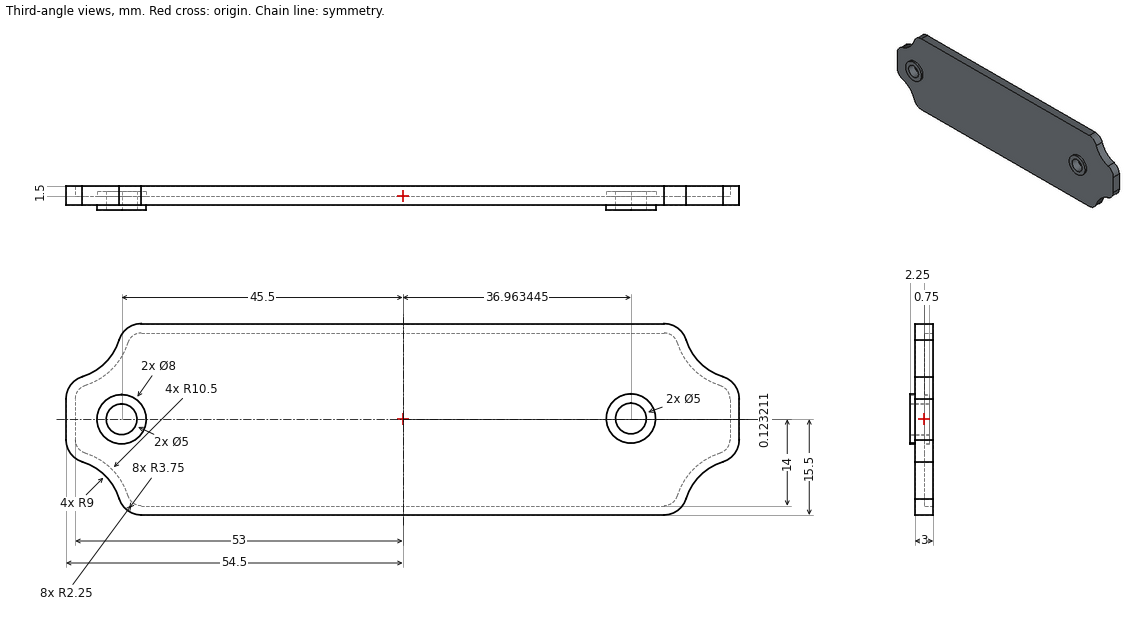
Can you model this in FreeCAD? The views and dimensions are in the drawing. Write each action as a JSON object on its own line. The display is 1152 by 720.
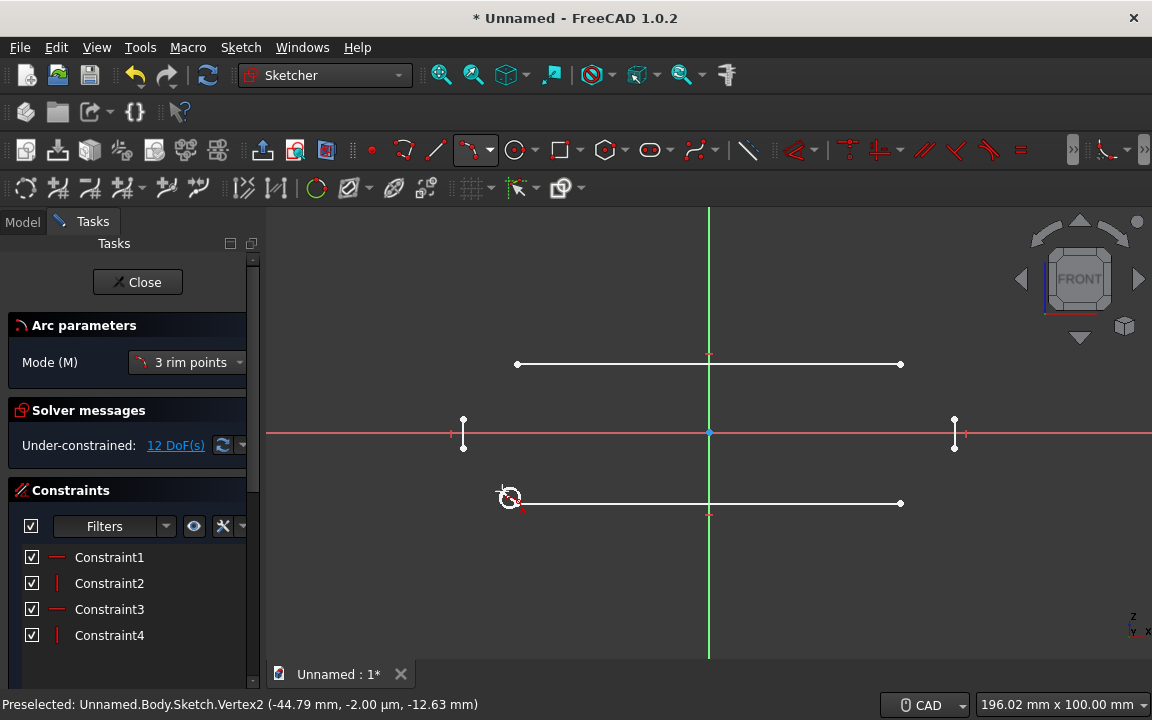
{"action": "scroll", "coordinate": [508, 500], "scroll_direction": "up", "scroll_amount": 8}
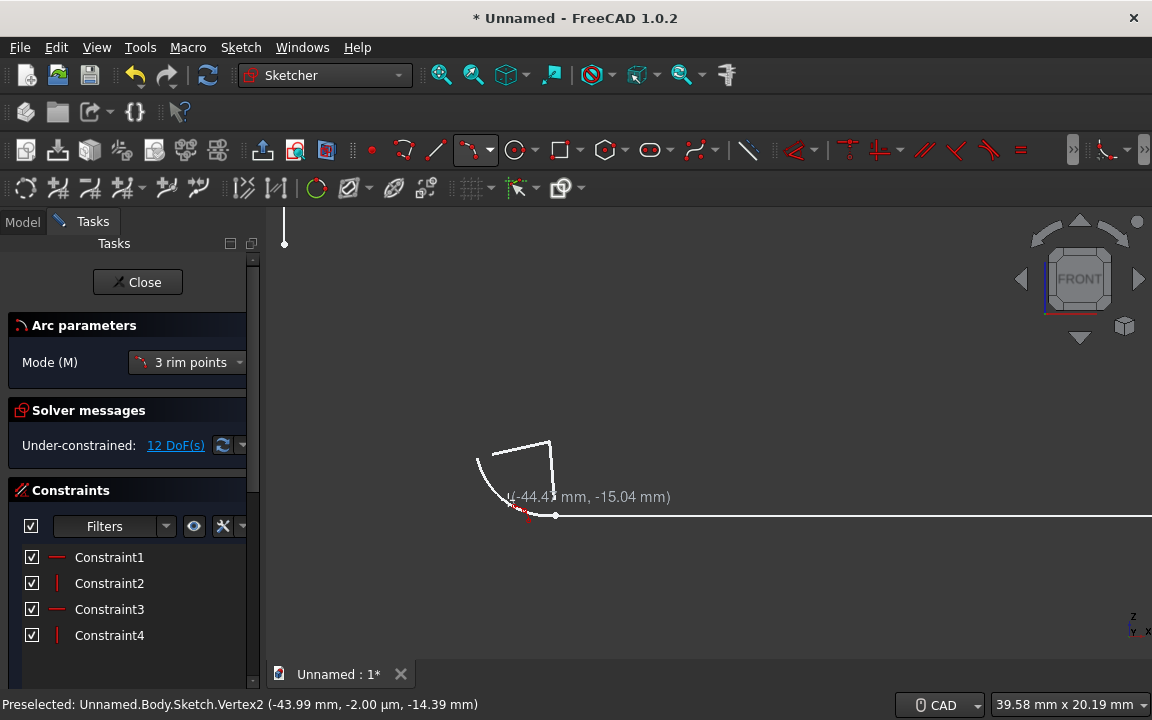
{"action": "left_click", "coordinate": [505, 496]}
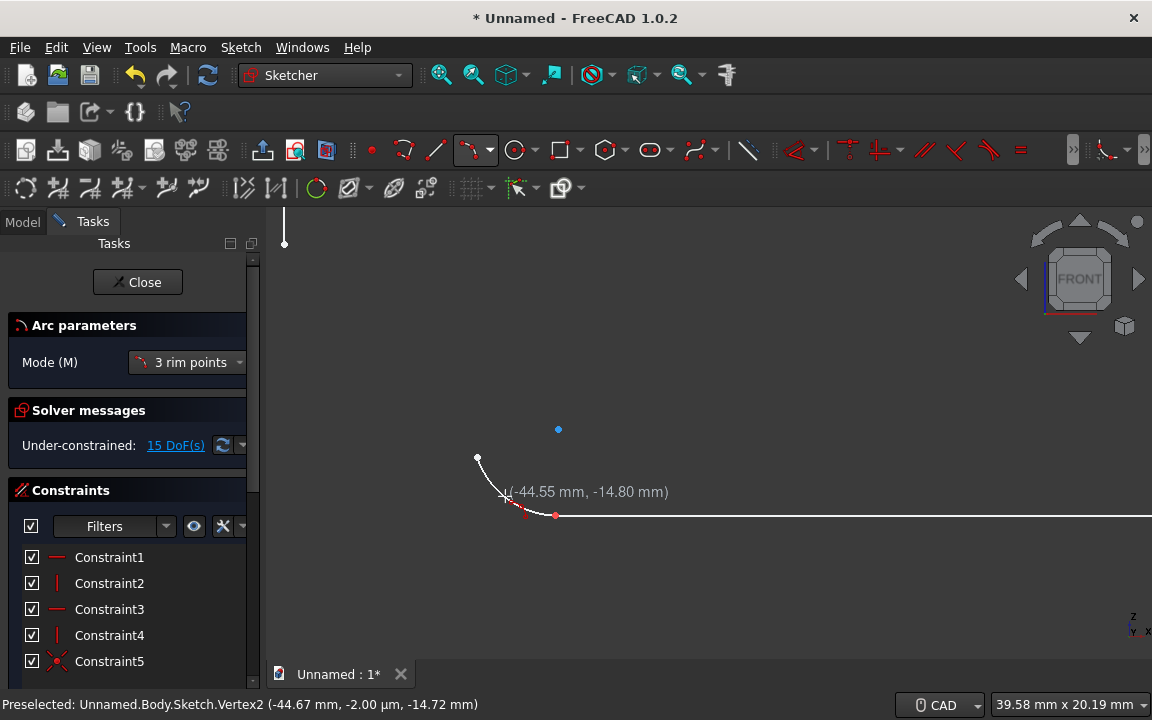
{"action": "scroll", "coordinate": [422, 501], "scroll_direction": "down", "scroll_amount": 8}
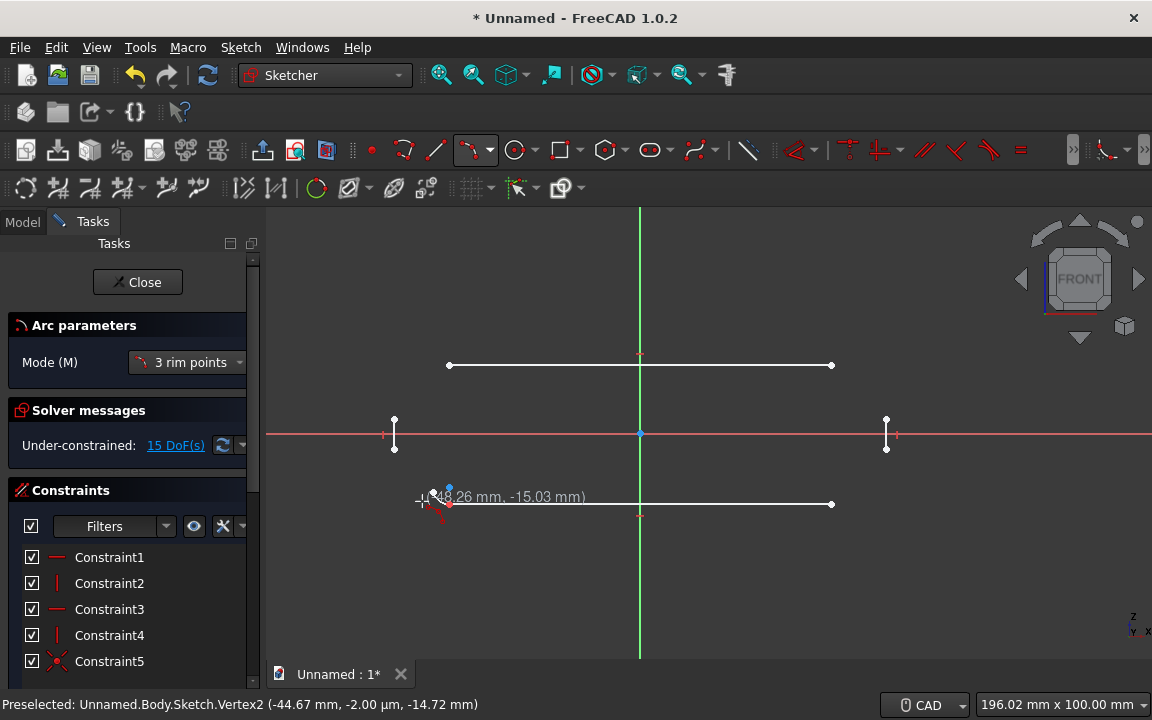
{"action": "left_click", "coordinate": [433, 493]}
{"action": "left_click", "coordinate": [406, 465]}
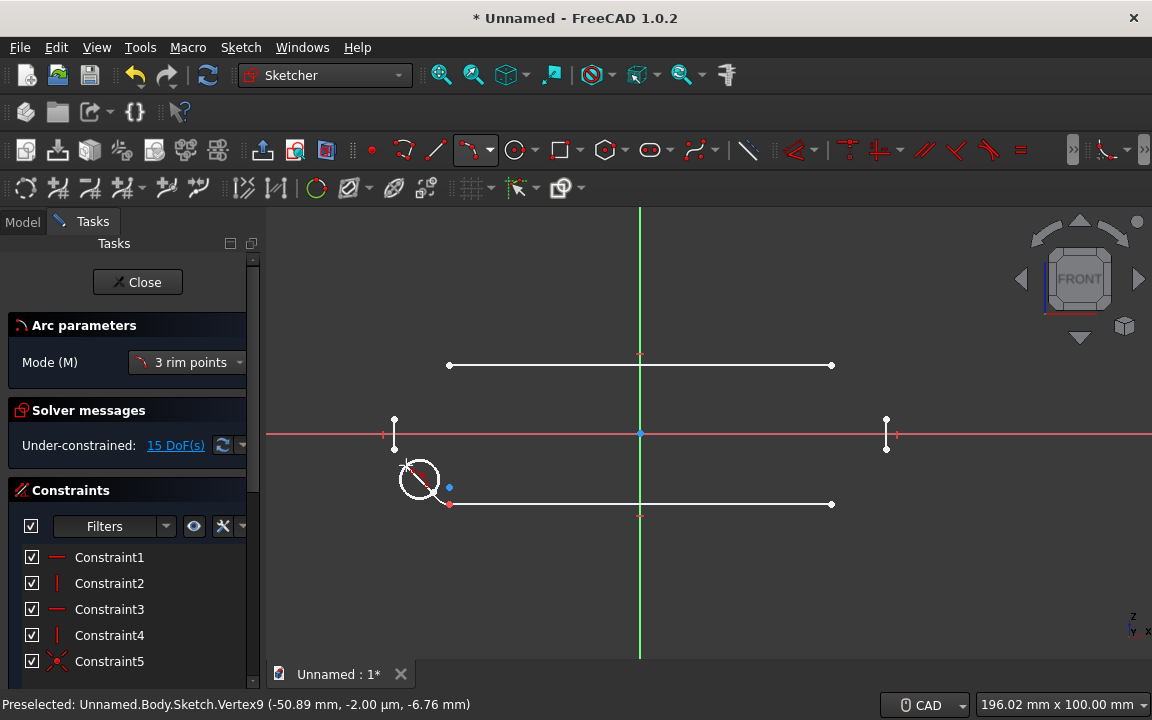
{"action": "scroll", "coordinate": [423, 475], "scroll_direction": "up", "scroll_amount": 7}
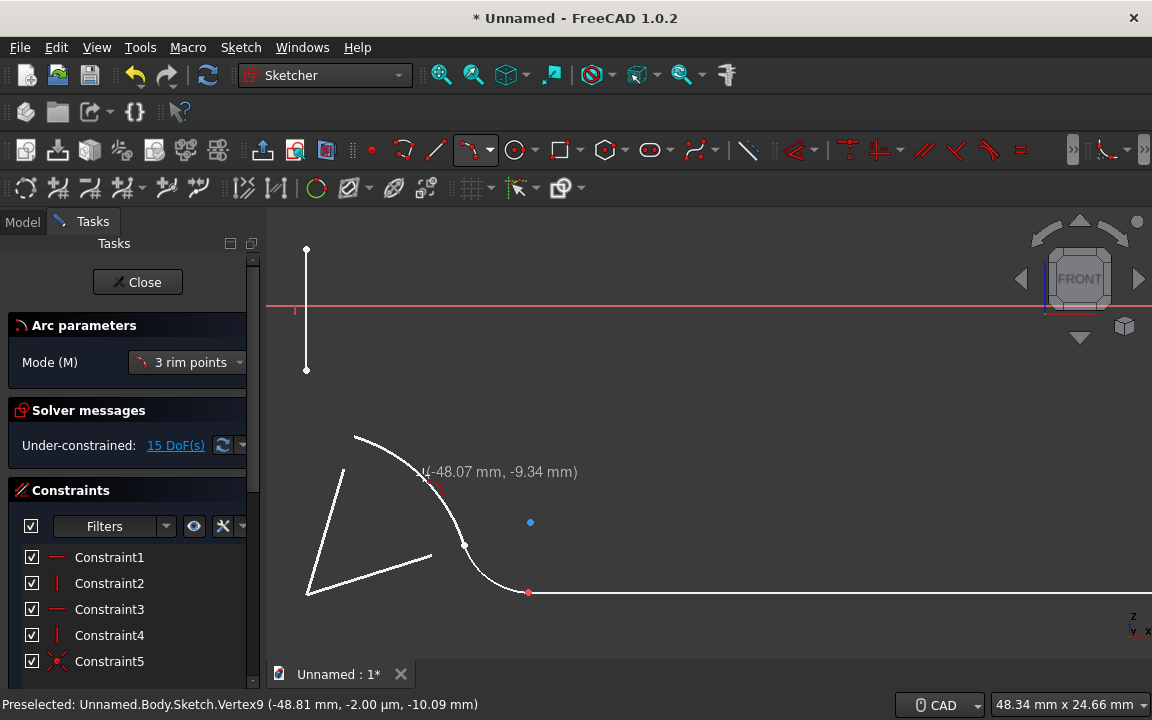
{"action": "left_click", "coordinate": [421, 474]}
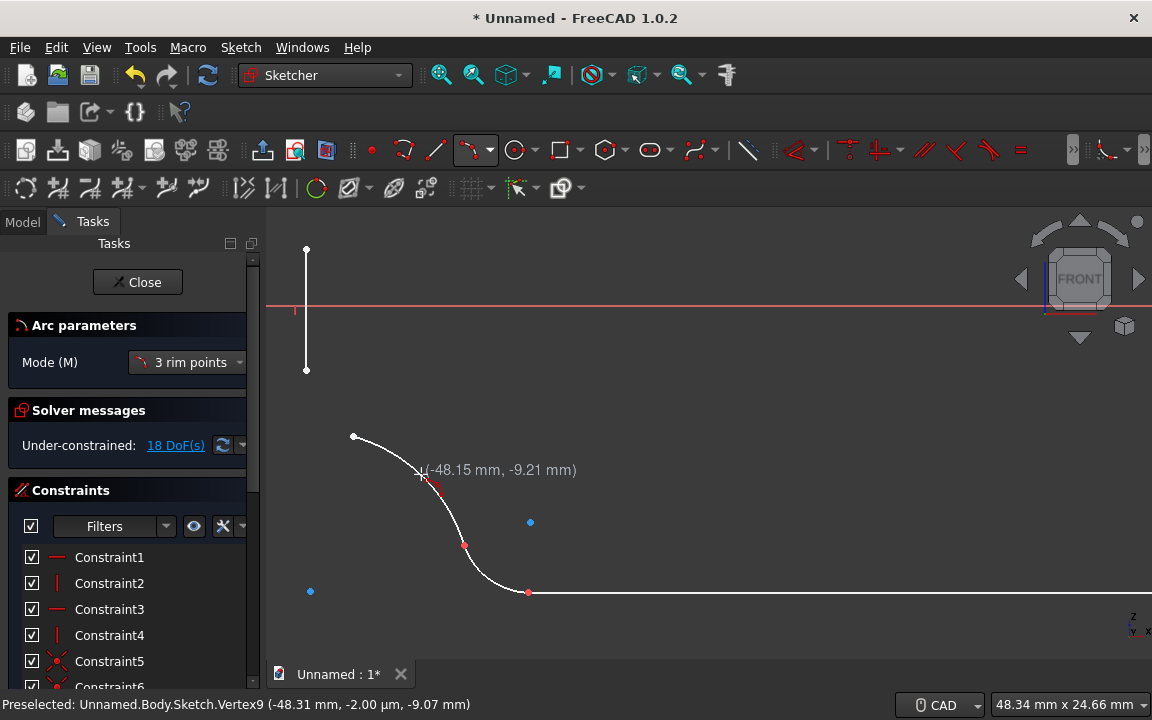
{"action": "scroll", "coordinate": [423, 475], "scroll_direction": "down", "scroll_amount": 7}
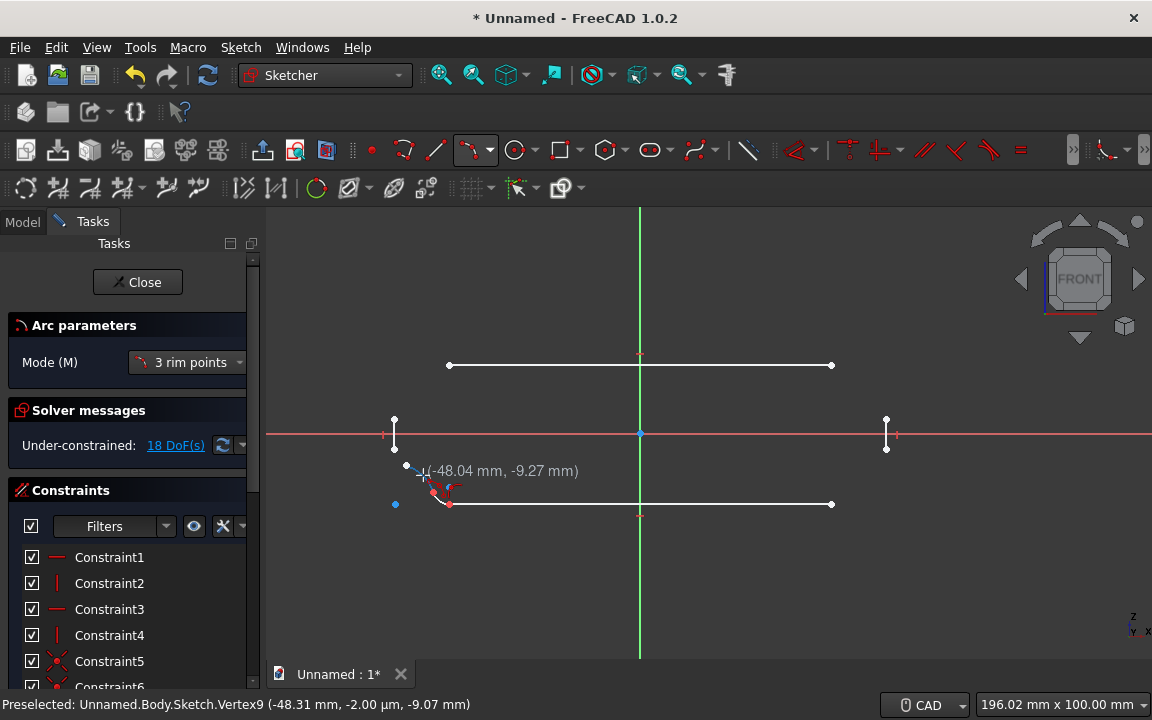
{"action": "left_click", "coordinate": [406, 466]}
{"action": "left_click", "coordinate": [394, 450]}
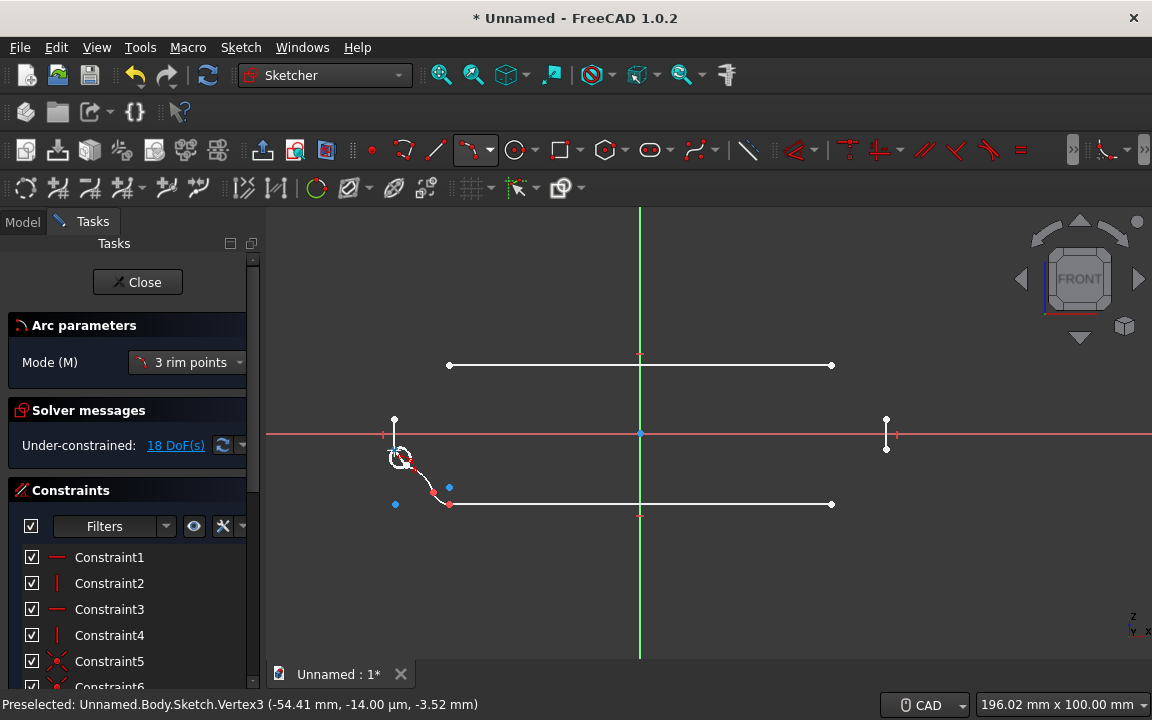
{"action": "scroll", "coordinate": [397, 459], "scroll_direction": "up", "scroll_amount": 8}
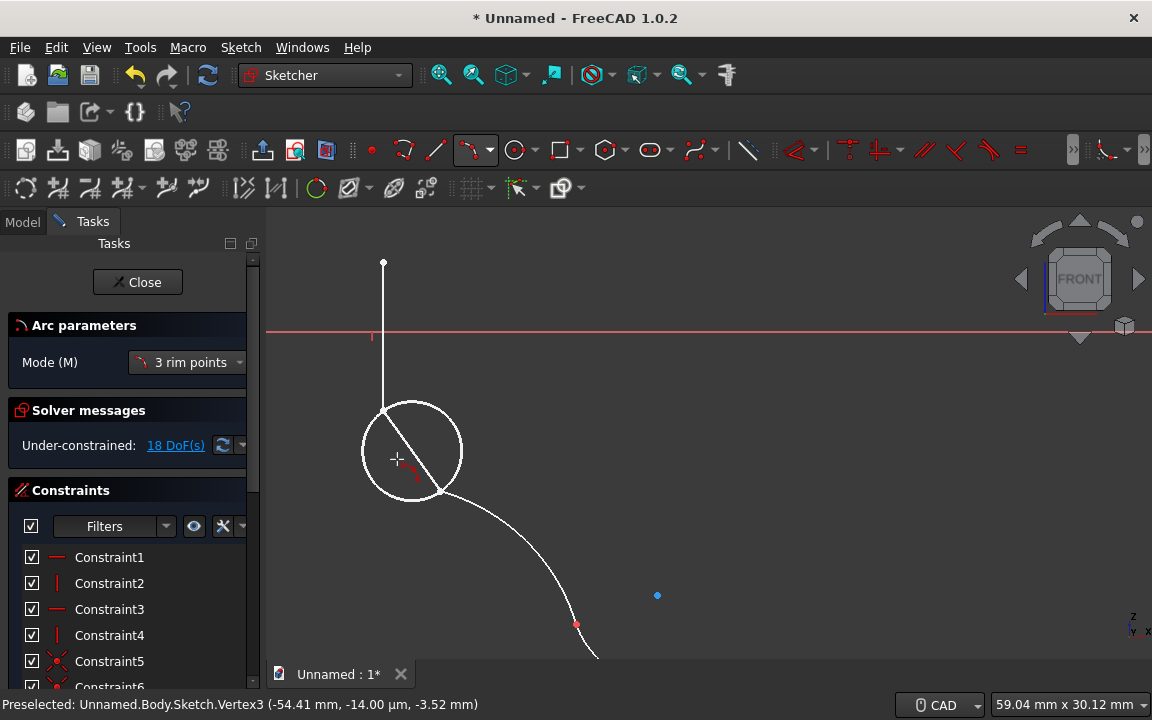
{"action": "left_click", "coordinate": [398, 456]}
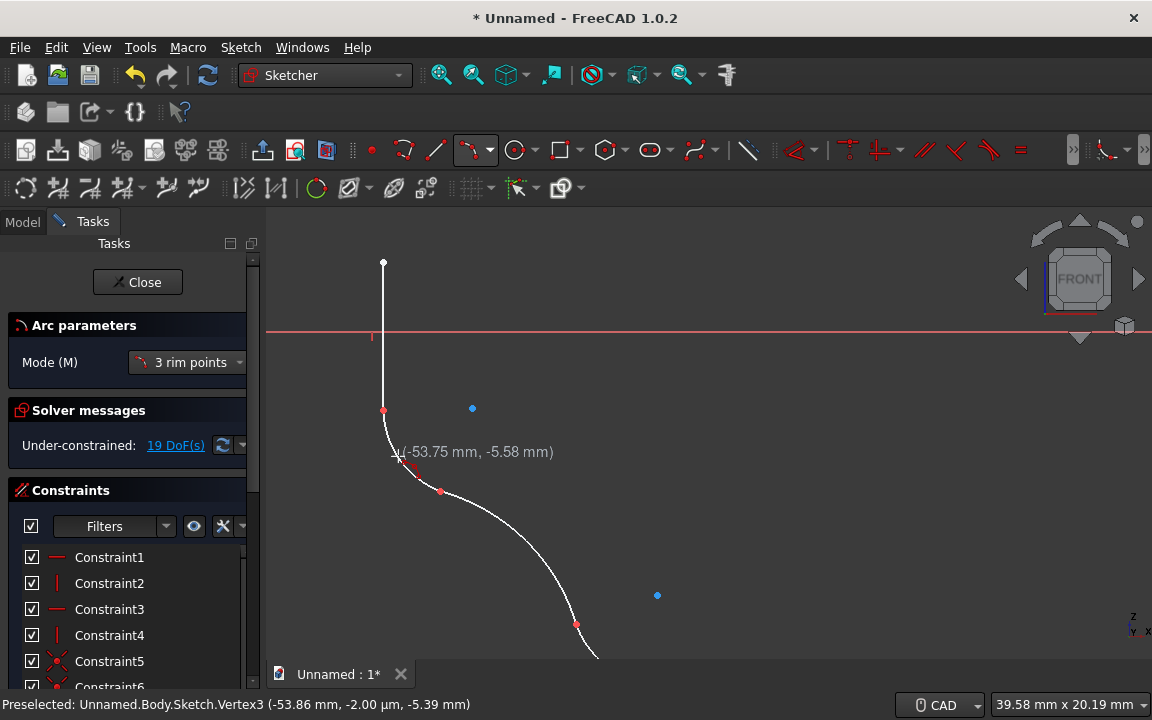
{"action": "scroll", "coordinate": [397, 459], "scroll_direction": "down", "scroll_amount": 8}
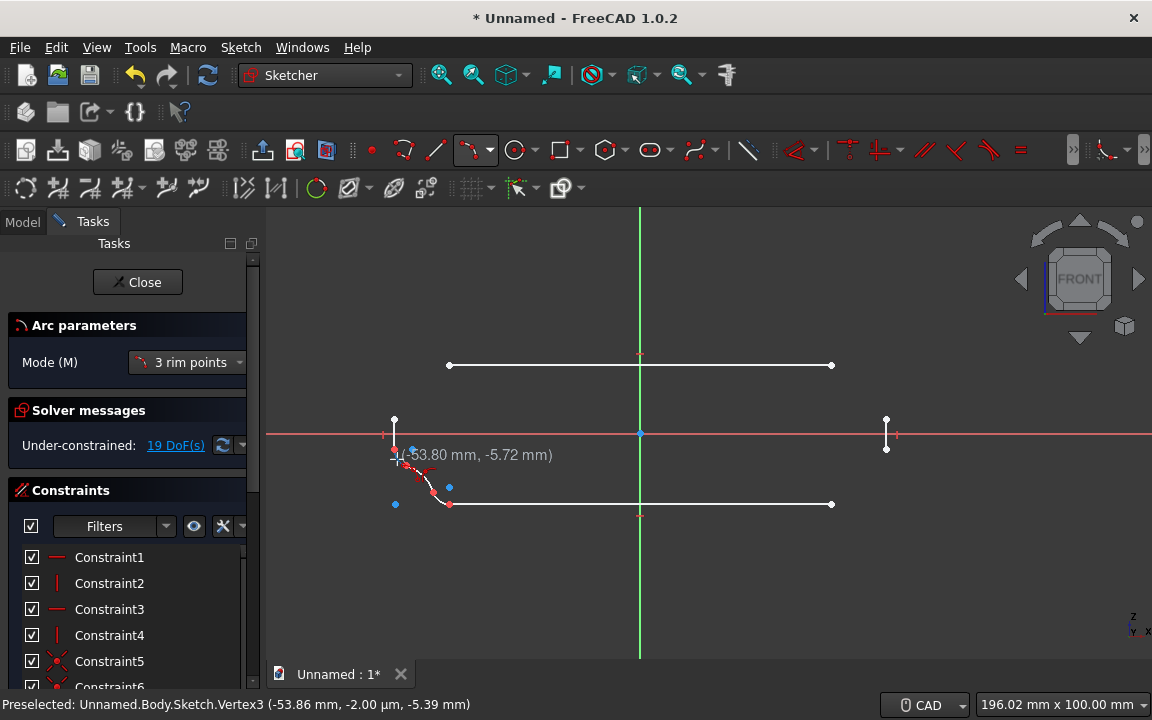
{"action": "left_click", "coordinate": [394, 420]}
{"action": "left_click", "coordinate": [406, 403]}